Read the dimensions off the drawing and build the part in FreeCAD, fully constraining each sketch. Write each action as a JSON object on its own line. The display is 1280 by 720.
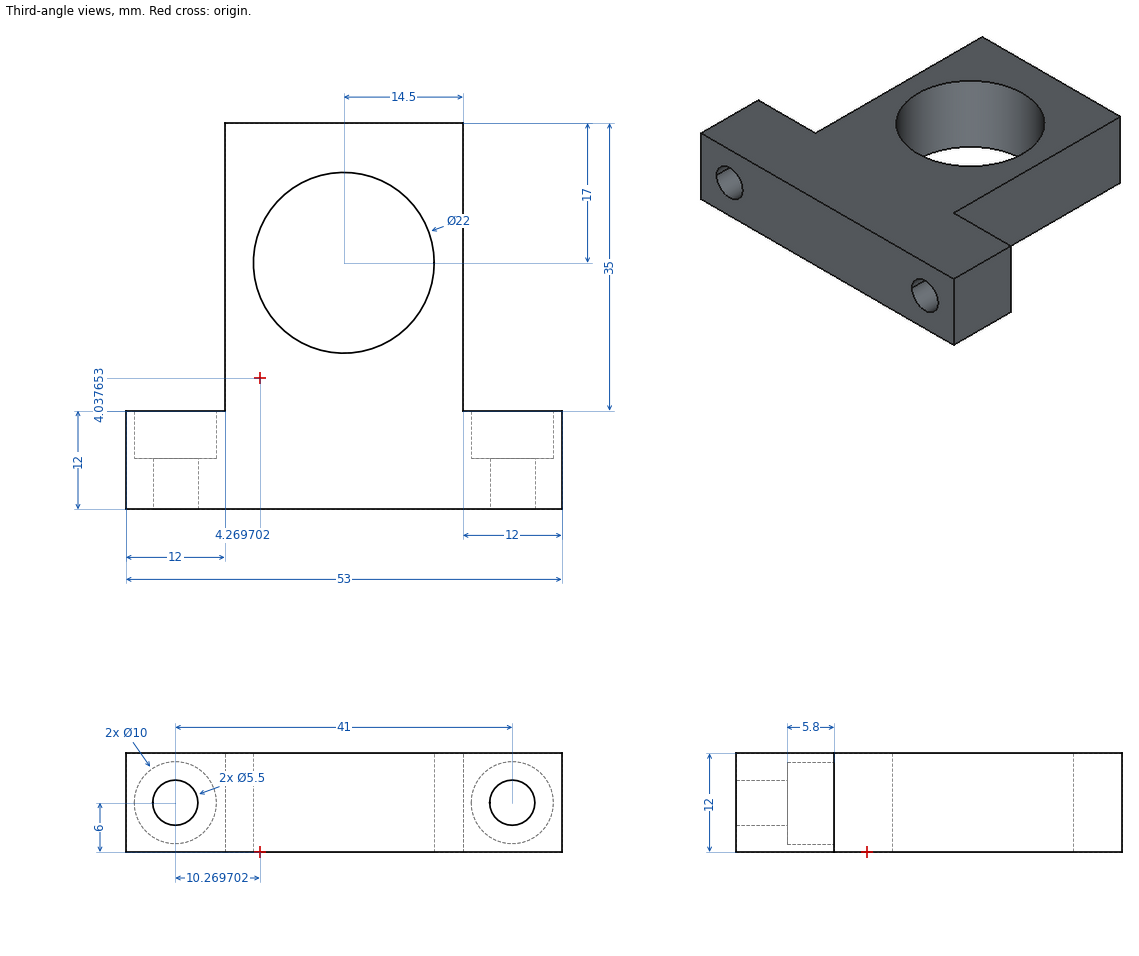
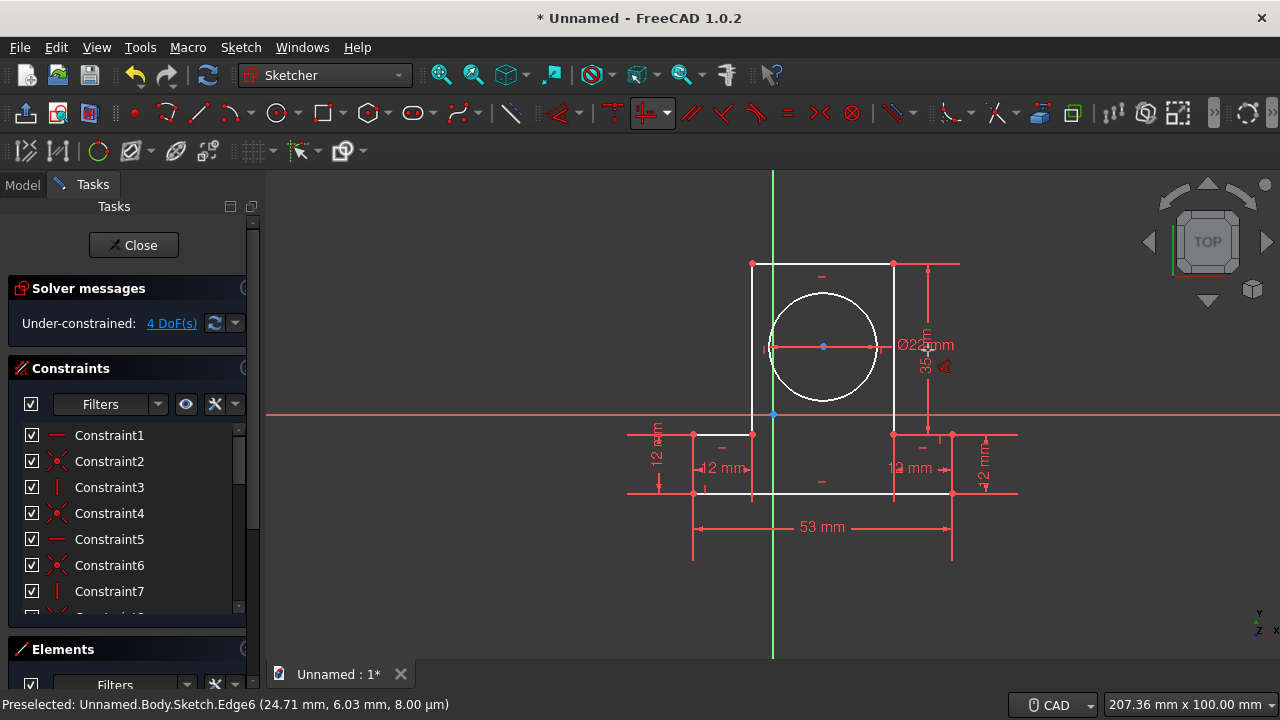
{"action": "left_click", "coordinate": [894, 264]}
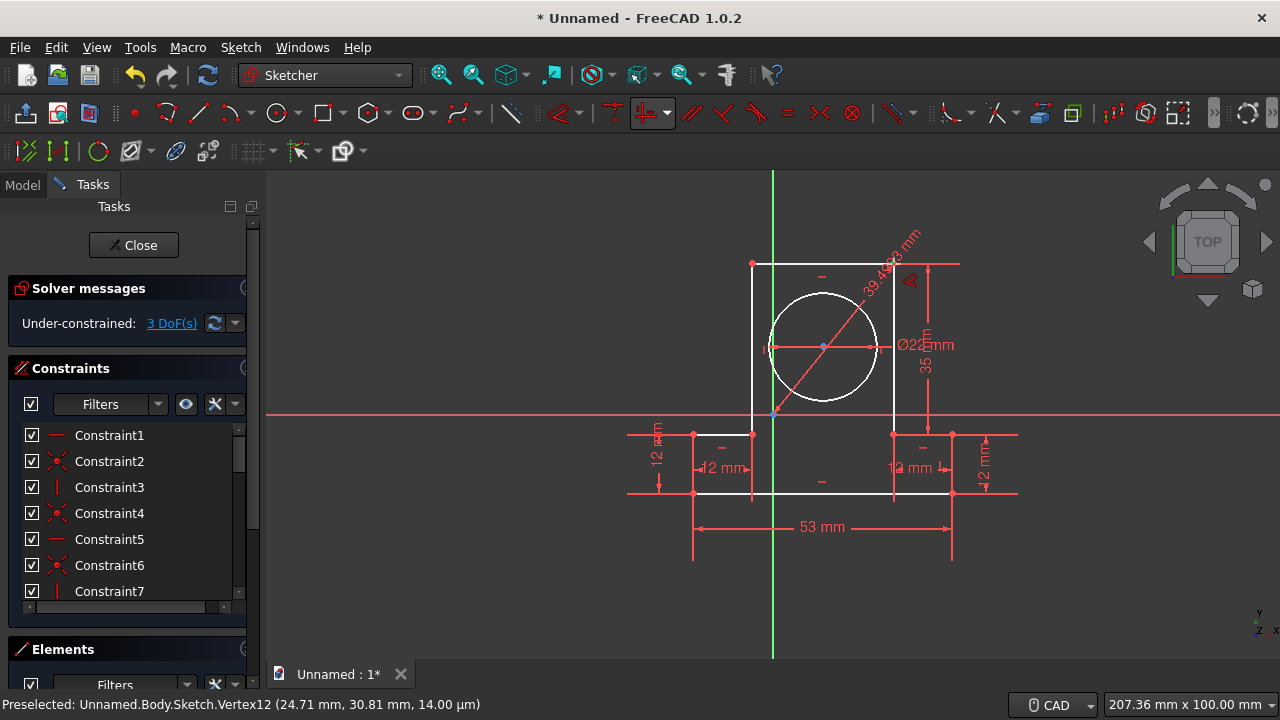
{"action": "left_click", "coordinate": [823, 347]}
{"action": "left_click", "coordinate": [928, 305]}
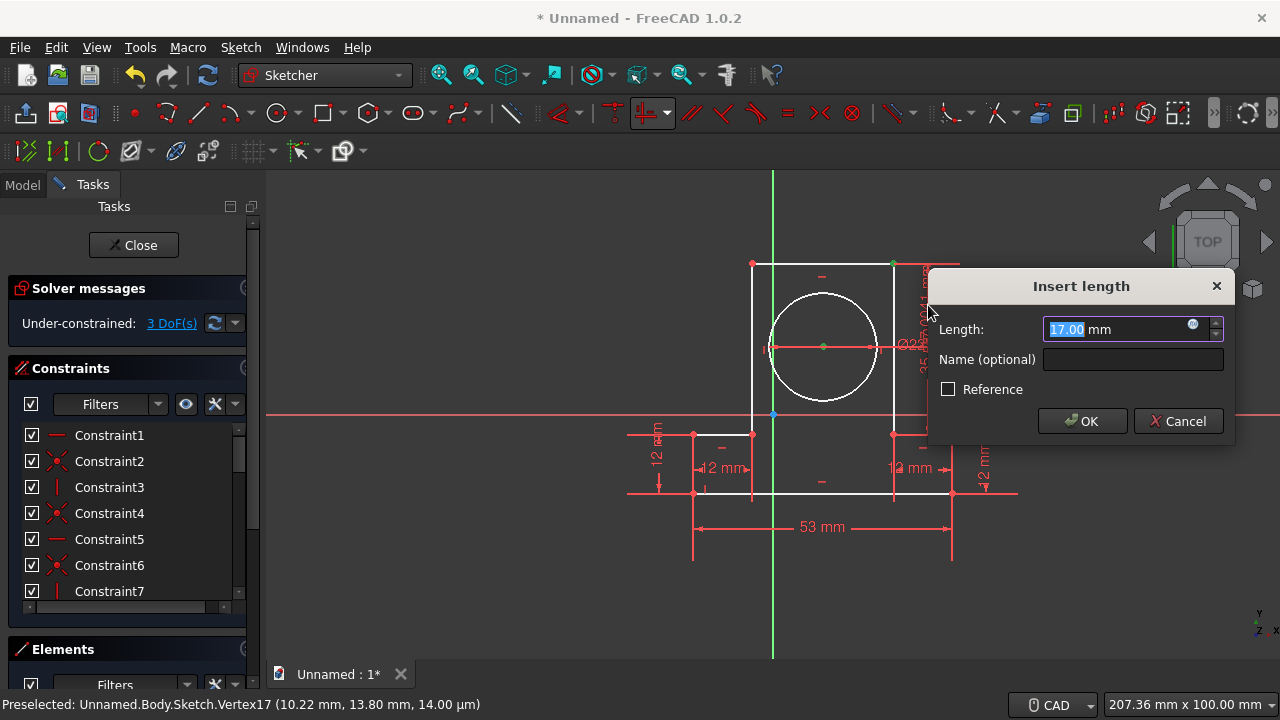
{"action": "type", "text": "17"}
{"action": "key", "text": "Return"}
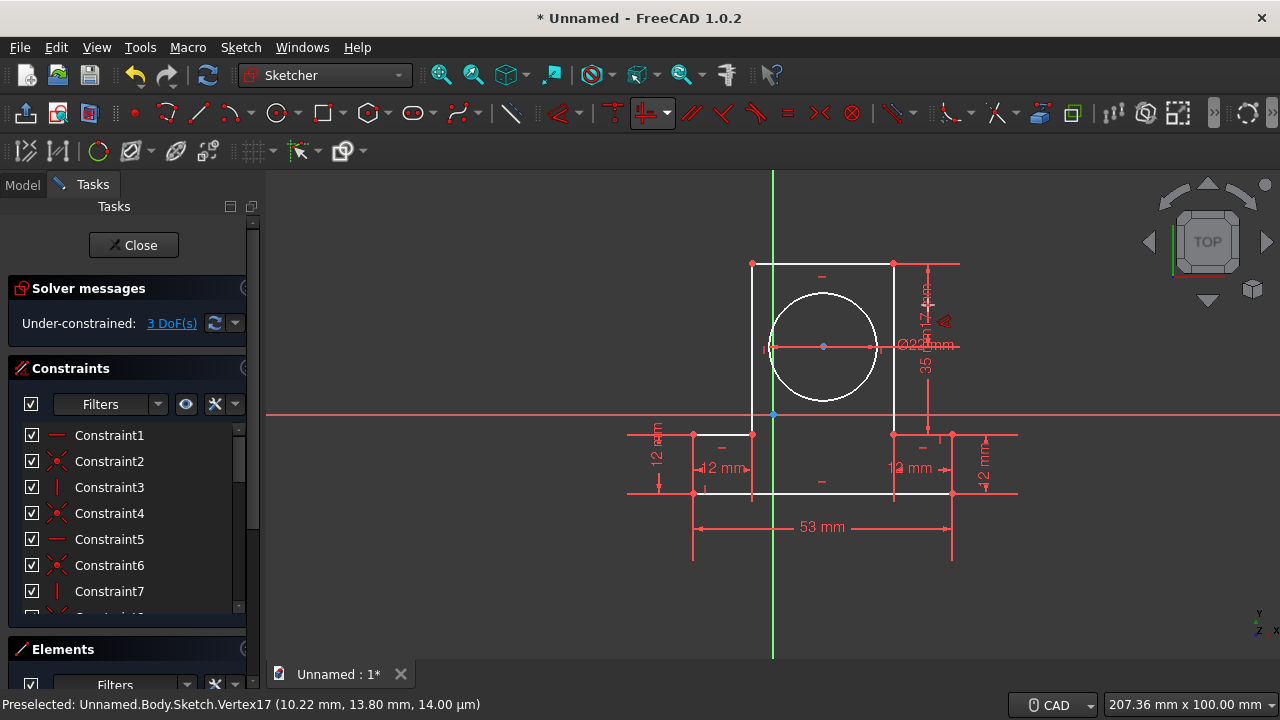
{"action": "left_click", "coordinate": [894, 264]}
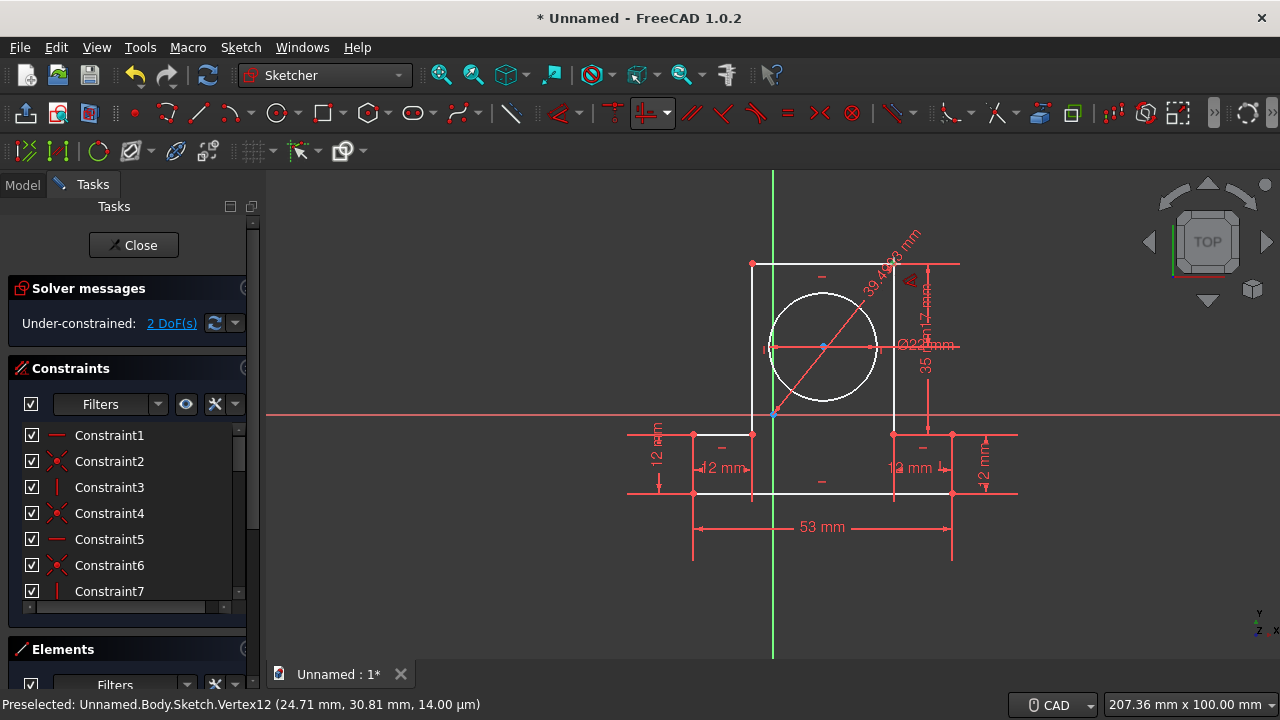
{"action": "left_click", "coordinate": [823, 347]}
{"action": "left_click", "coordinate": [858, 230]}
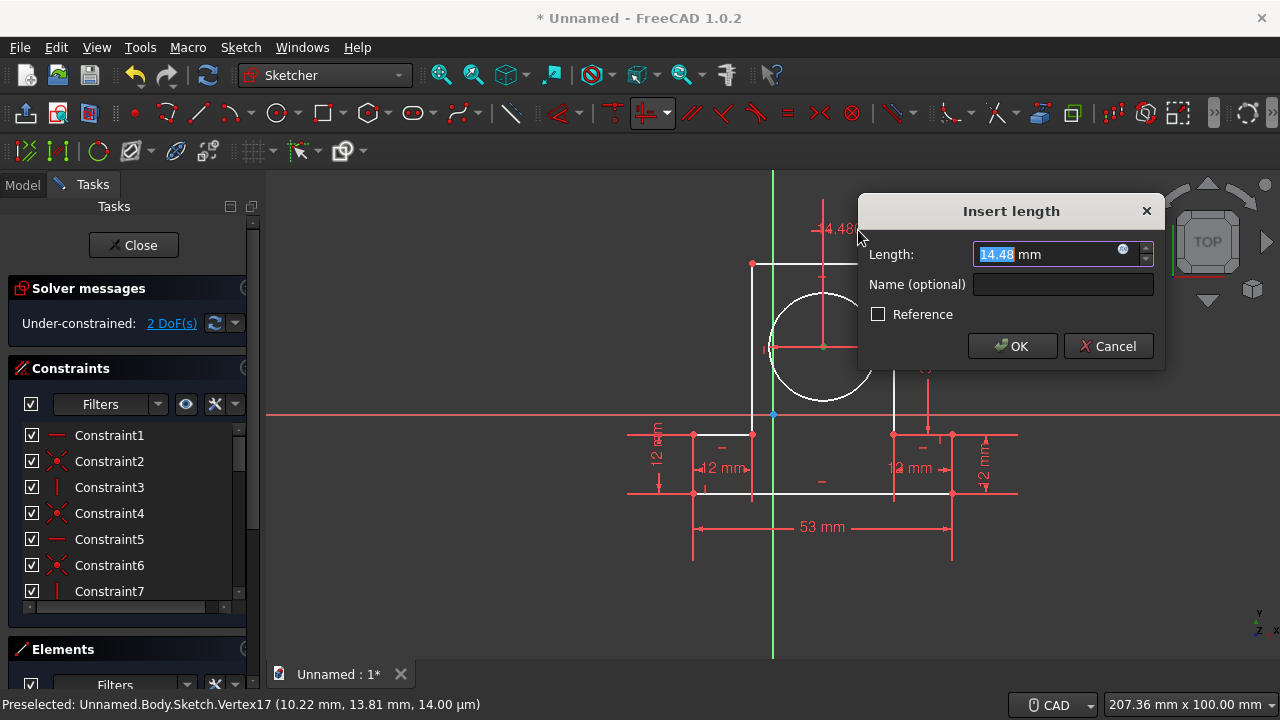
{"action": "type", "text": "14.5"}
{"action": "key", "text": "Return"}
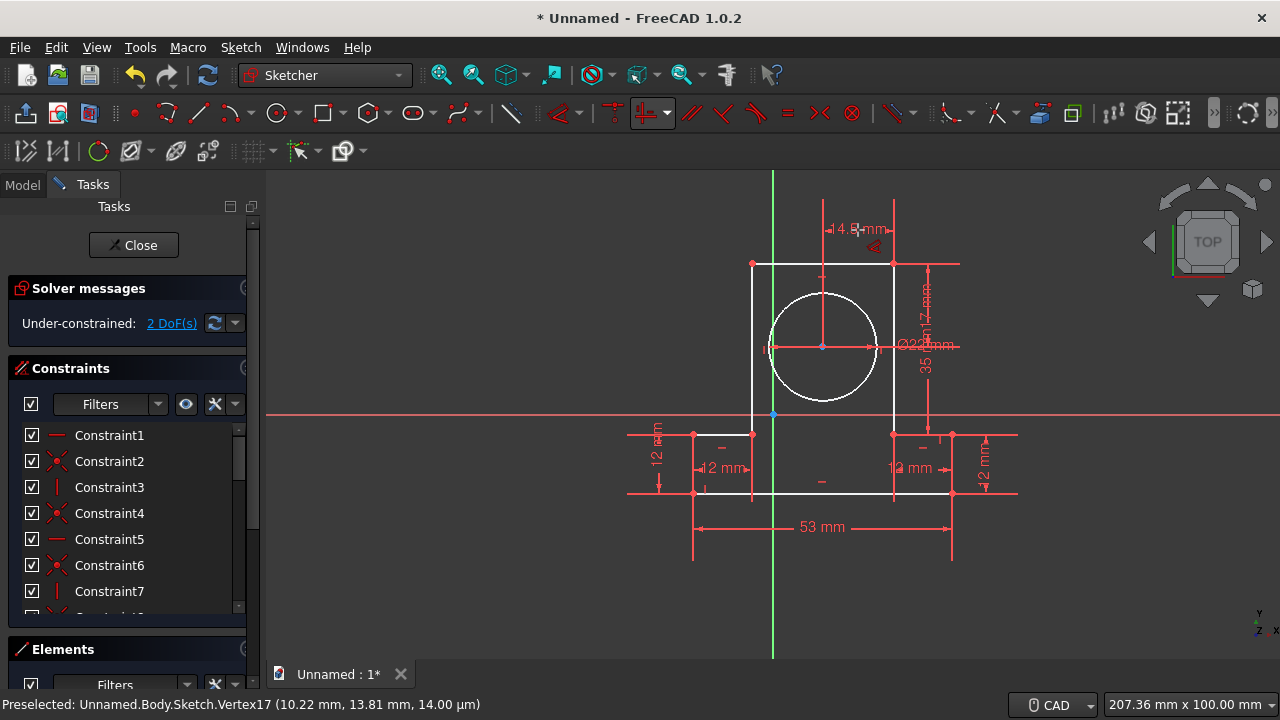
{"action": "scroll", "coordinate": [752, 435], "scroll_direction": "up", "scroll_amount": 4}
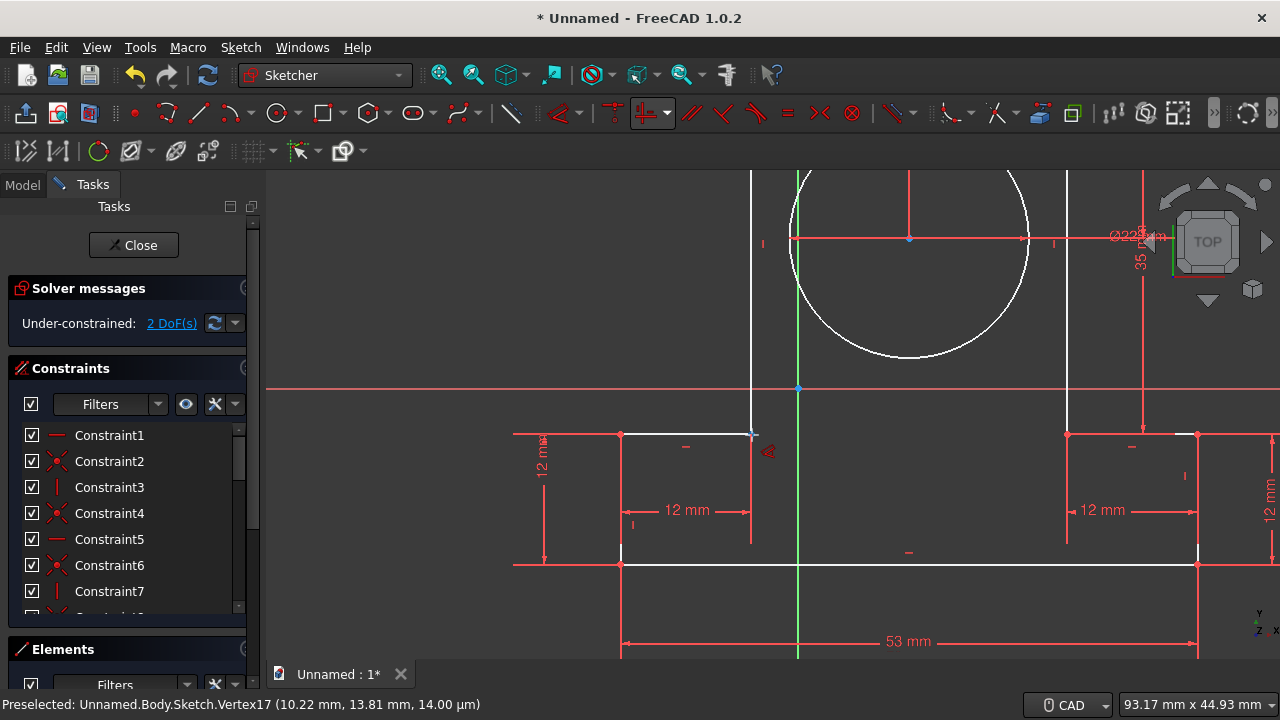
{"action": "left_click", "coordinate": [751, 434]}
{"action": "left_click", "coordinate": [775, 468]}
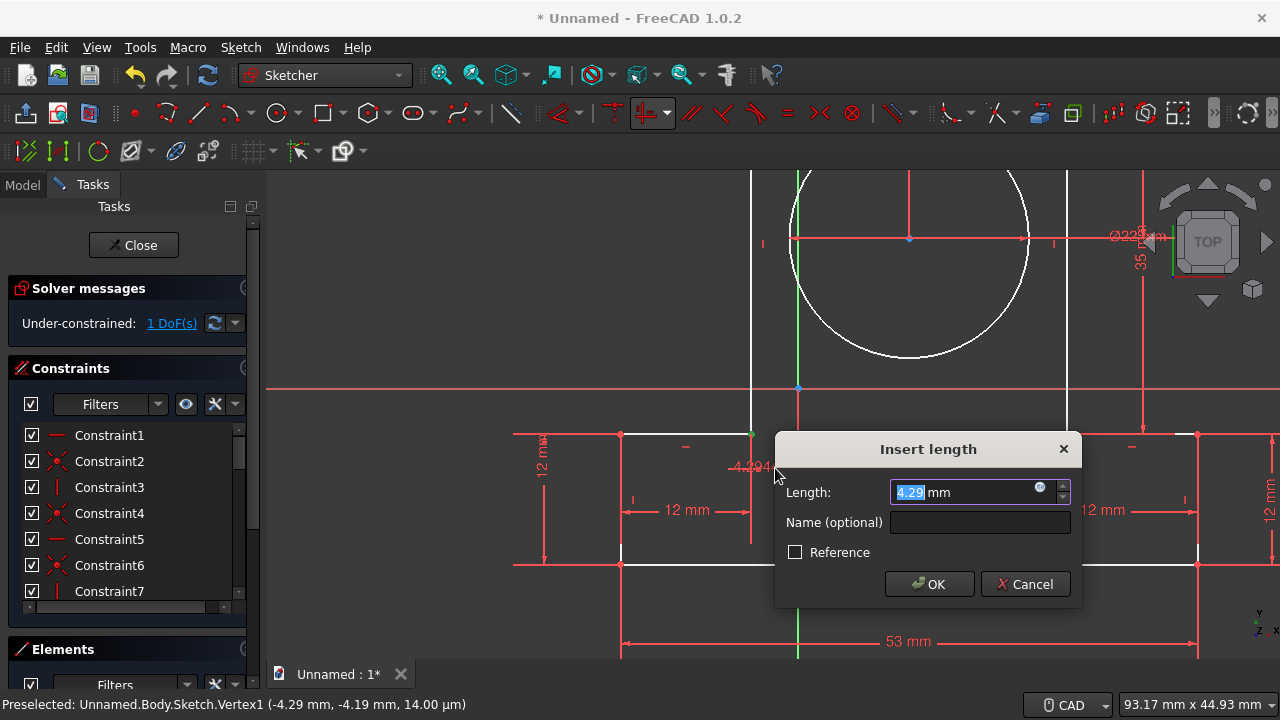
{"action": "type", "text": "4.269702"}
{"action": "key", "text": "Return"}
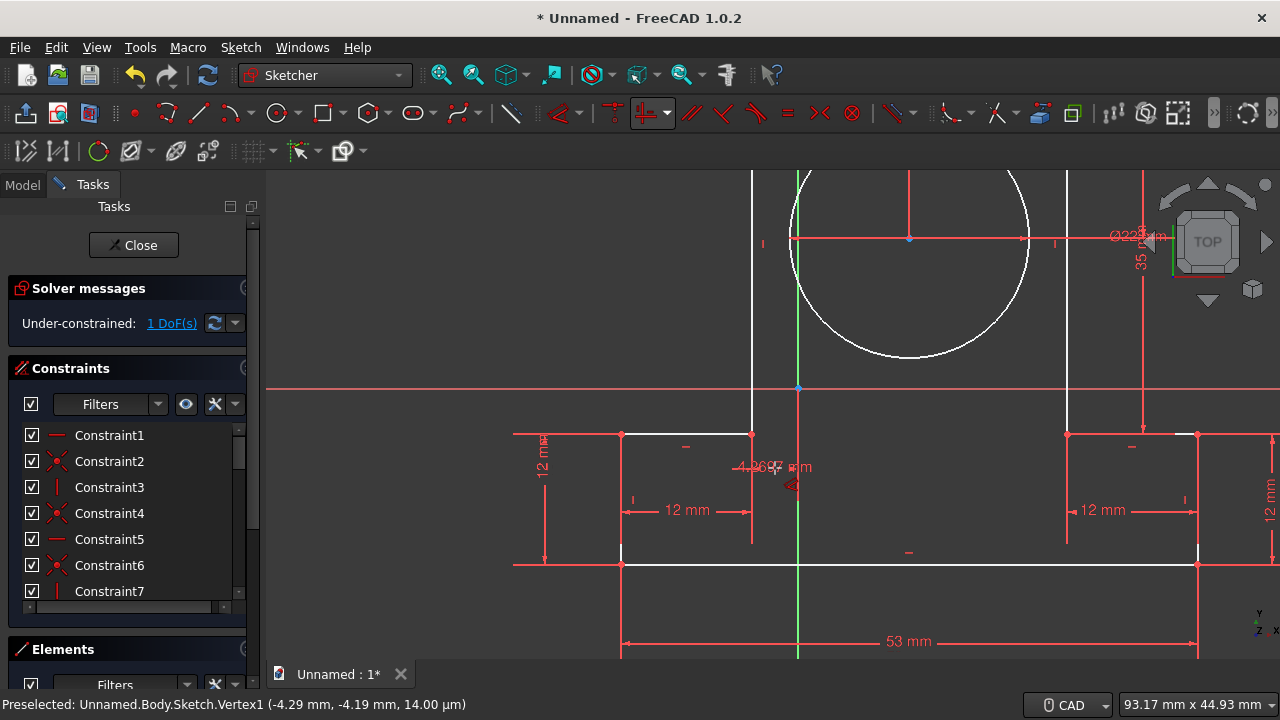
{"action": "left_click", "coordinate": [752, 434]}
{"action": "left_click", "coordinate": [718, 412]}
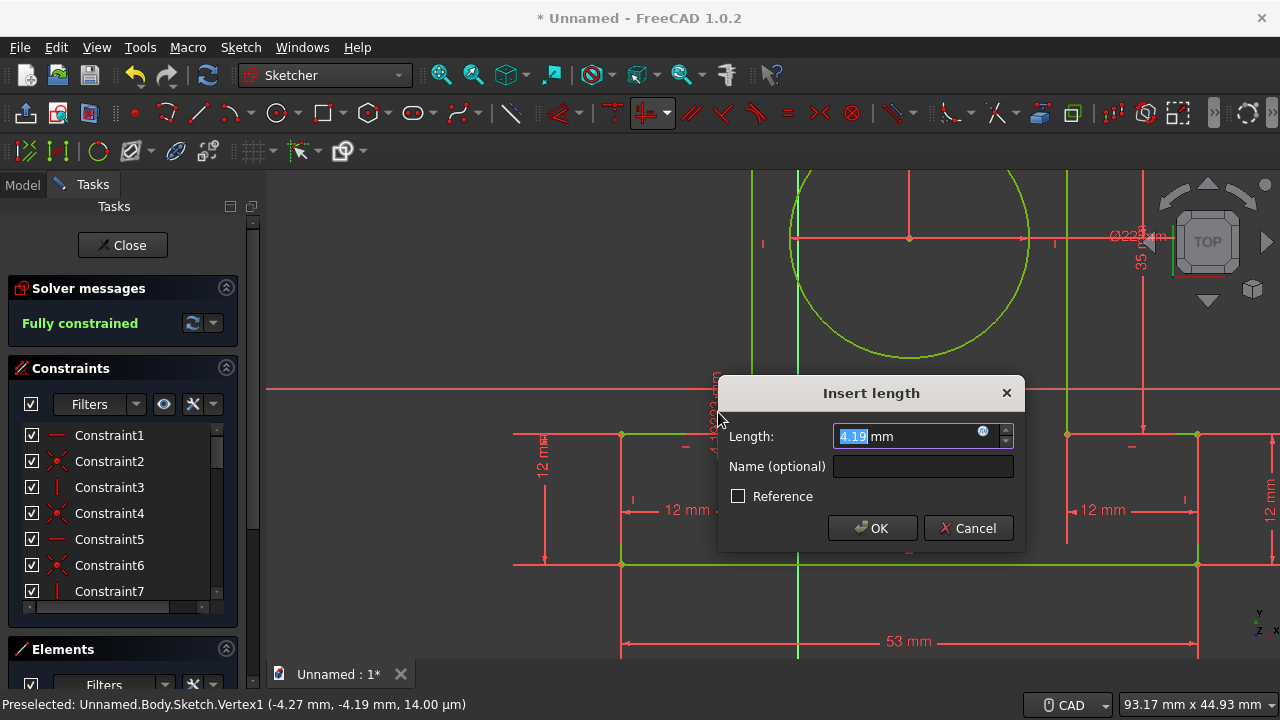
{"action": "type", "text": "4.037653"}
{"action": "key", "text": "Return"}
{"action": "key", "text": "Escape"}